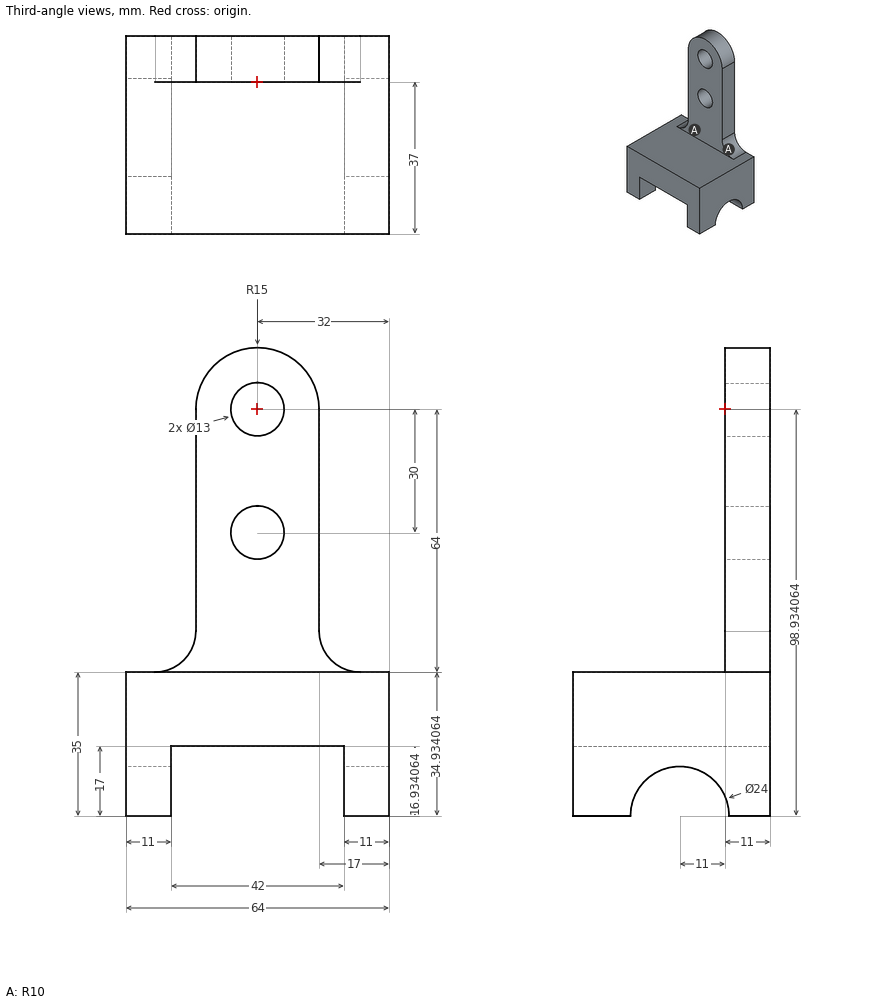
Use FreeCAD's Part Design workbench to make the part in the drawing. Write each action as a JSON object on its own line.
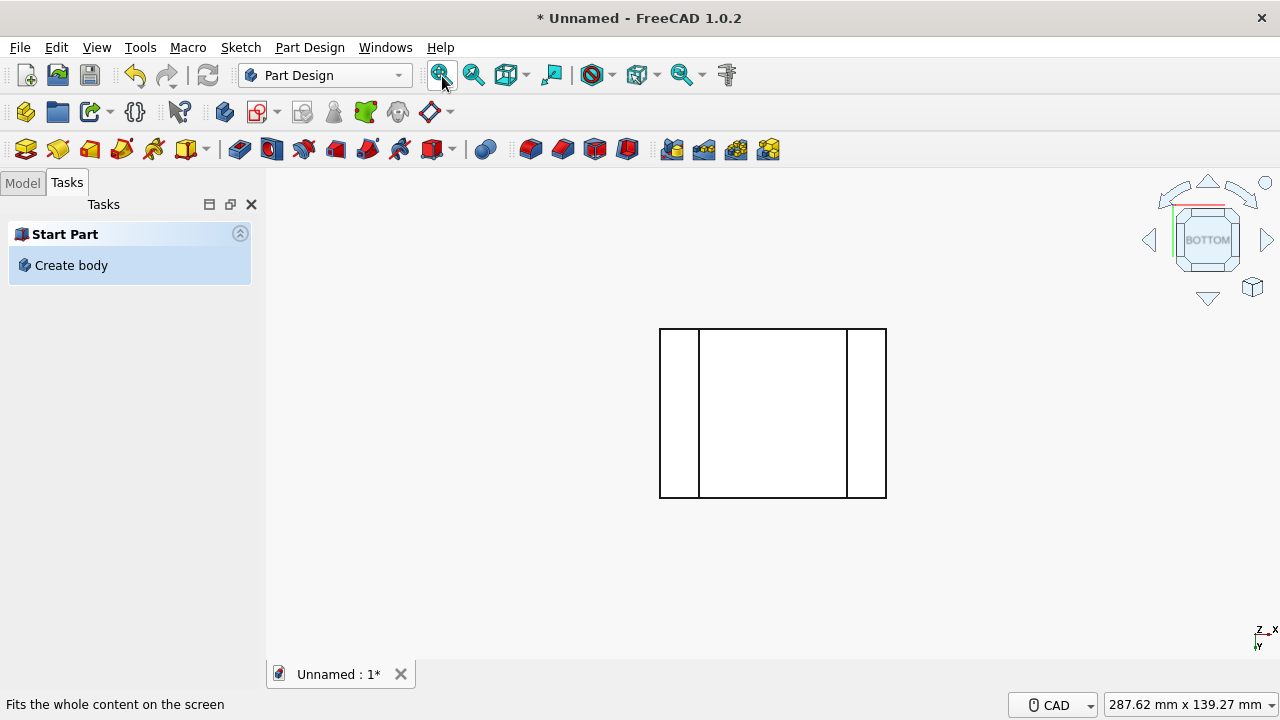
{"action": "key", "text": "4"}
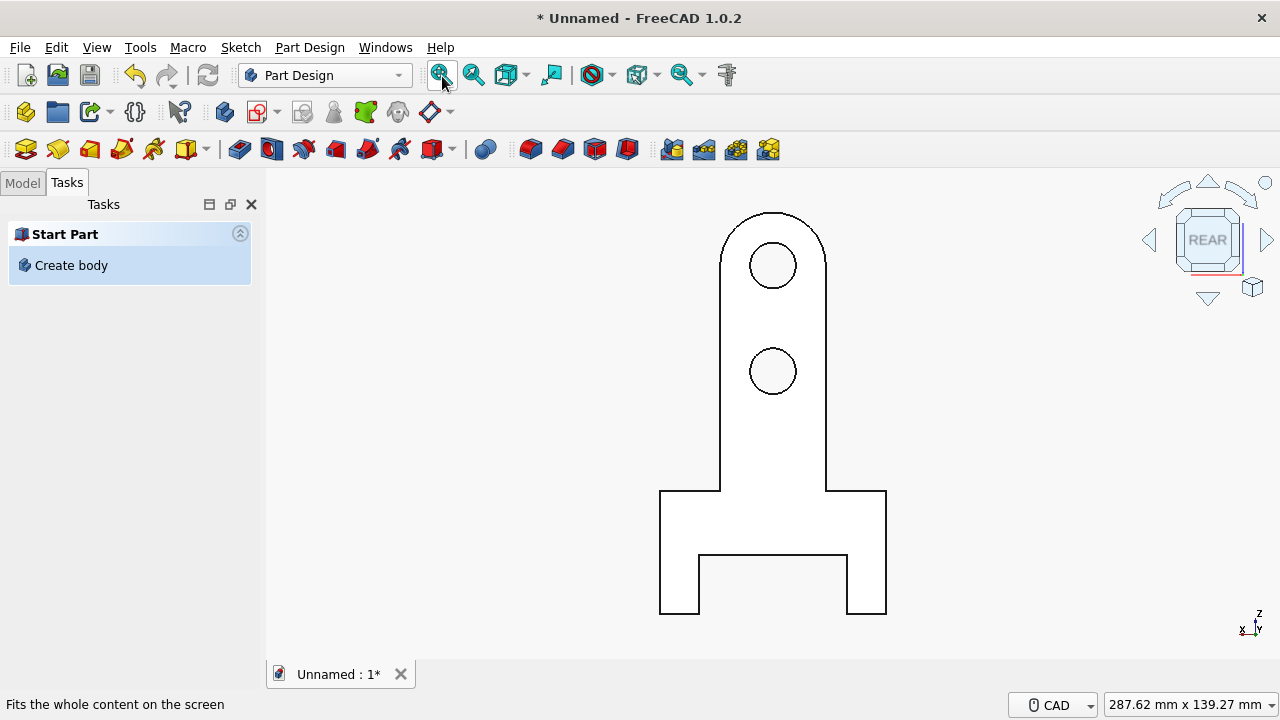
{"action": "key", "text": "6"}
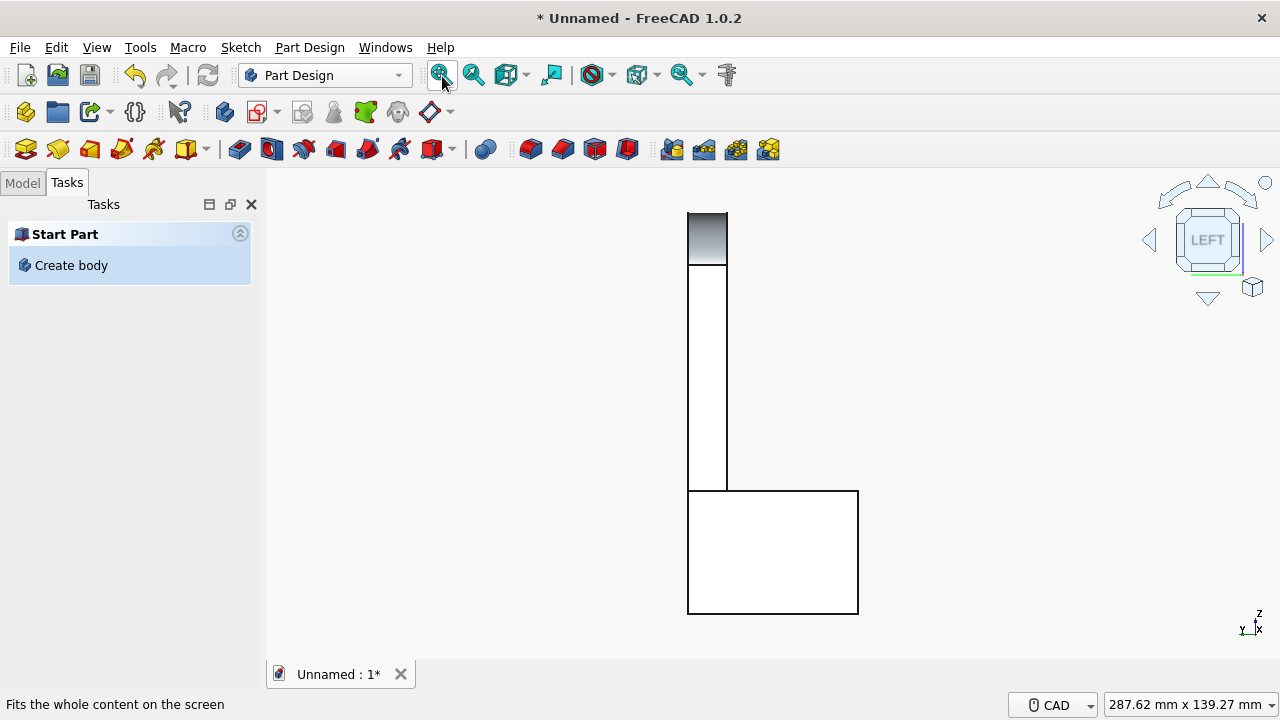
{"action": "key", "text": "v 3"}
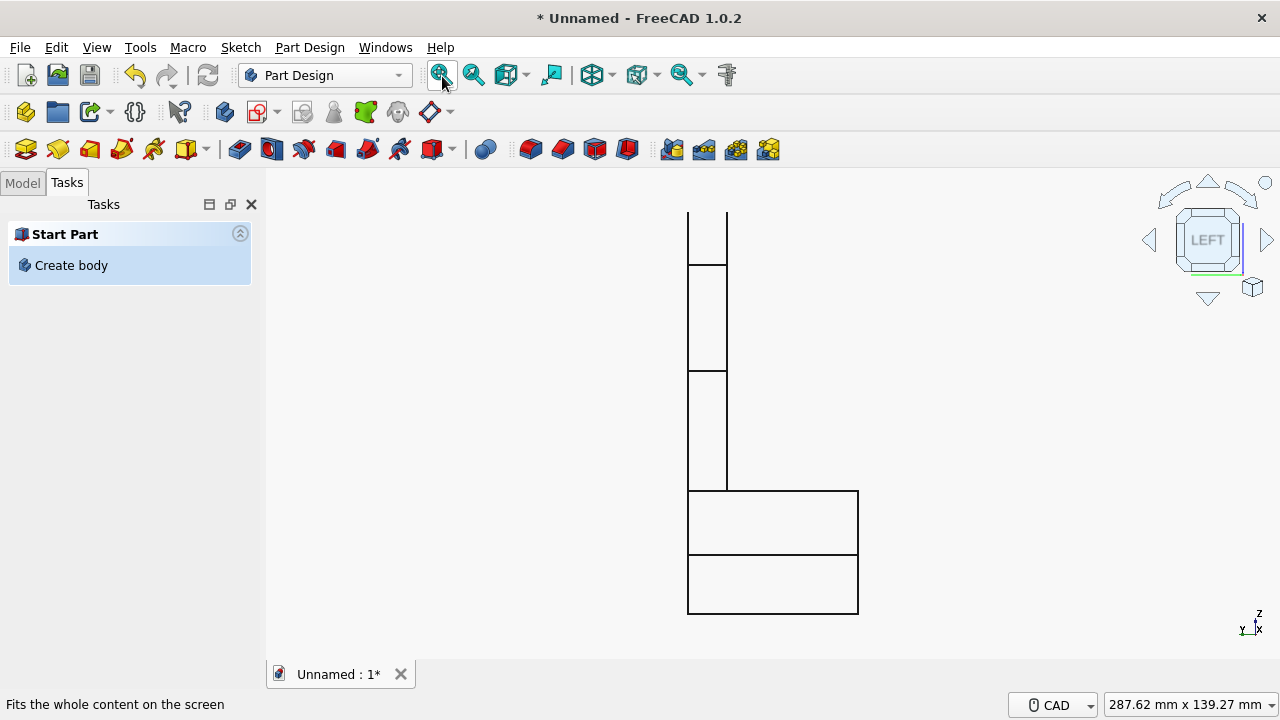
{"action": "key", "text": "0"}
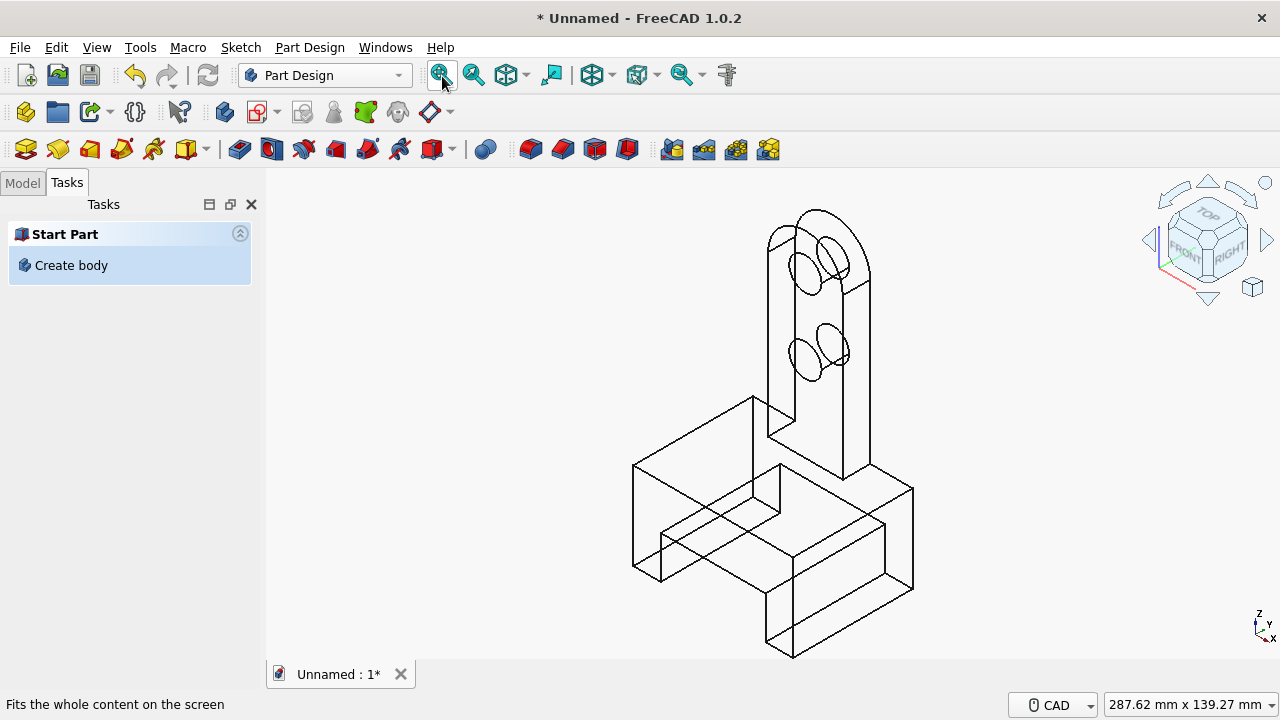
{"action": "left_click", "coordinate": [782, 428]}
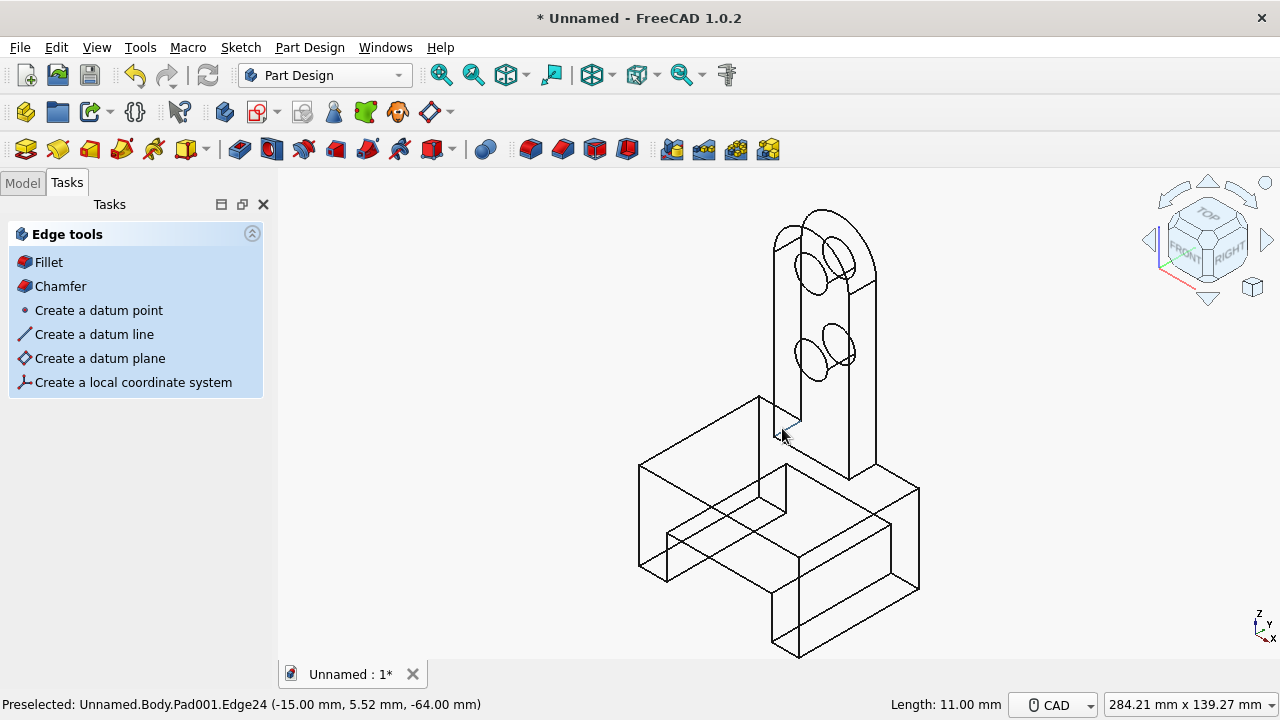
{"action": "left_click", "coordinate": [863, 471], "text": "ctrl"}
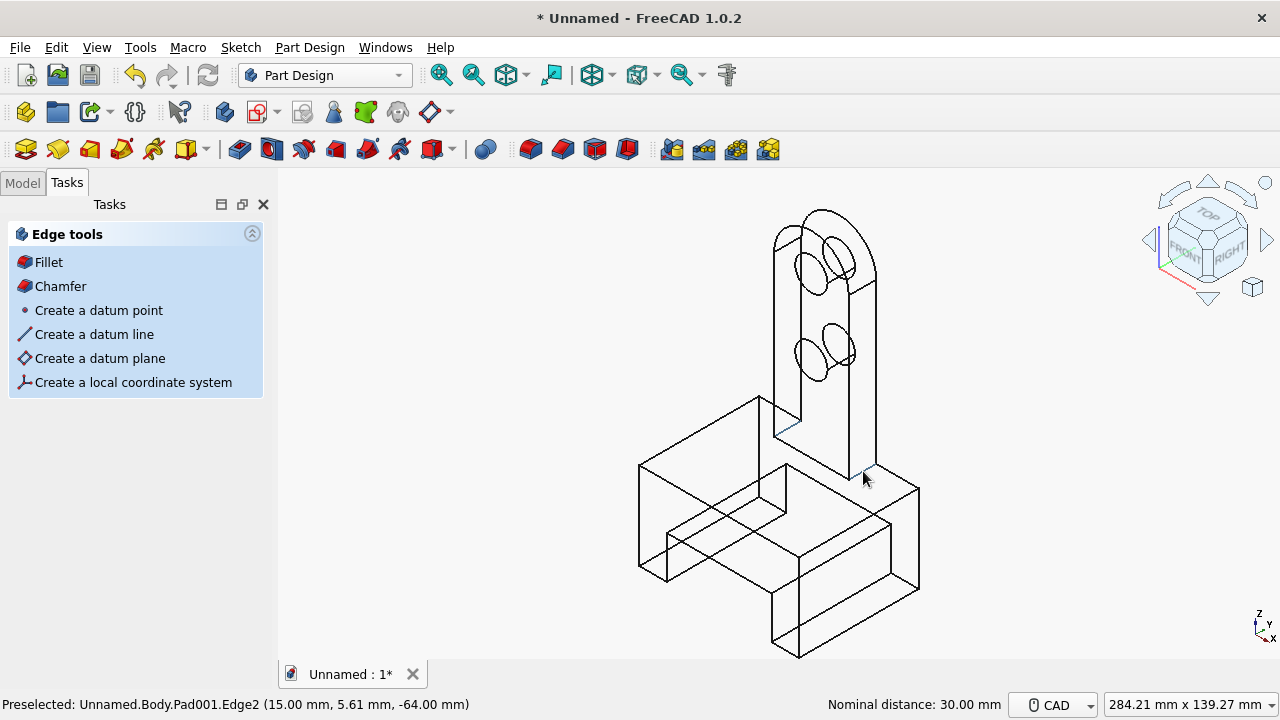
{"action": "key", "text": "v 1"}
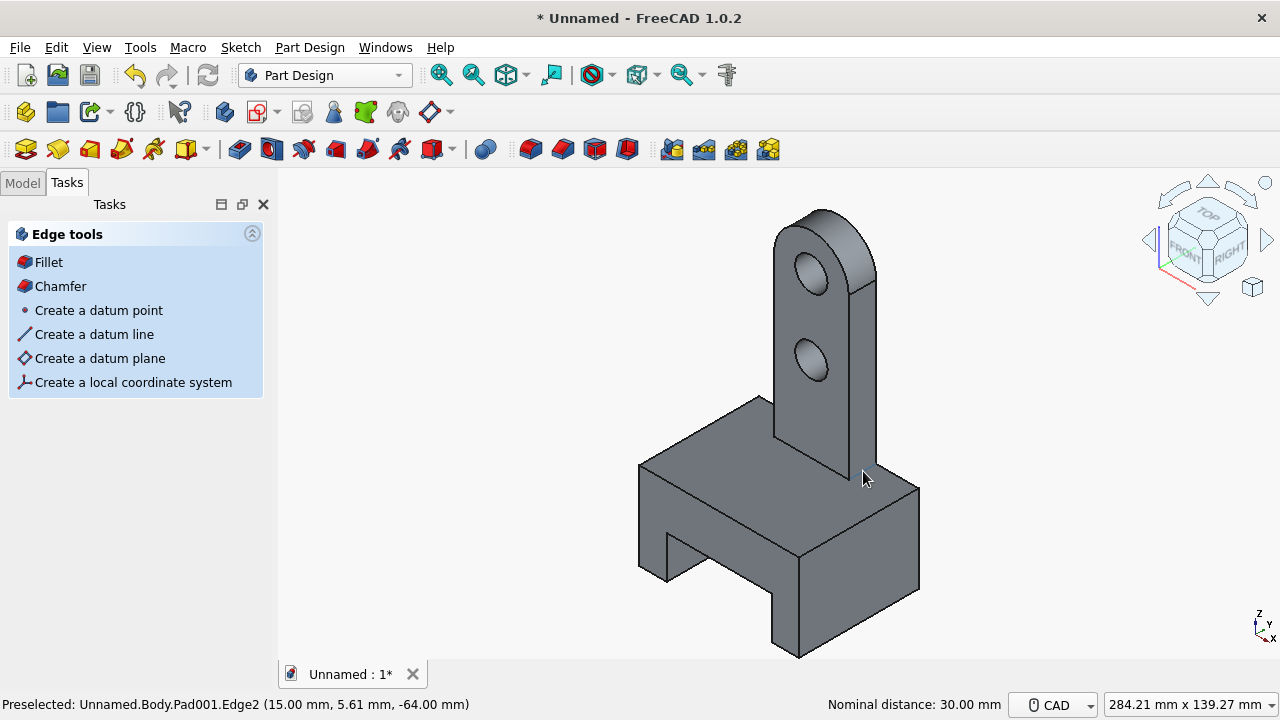
{"action": "left_click", "coordinate": [532, 150]}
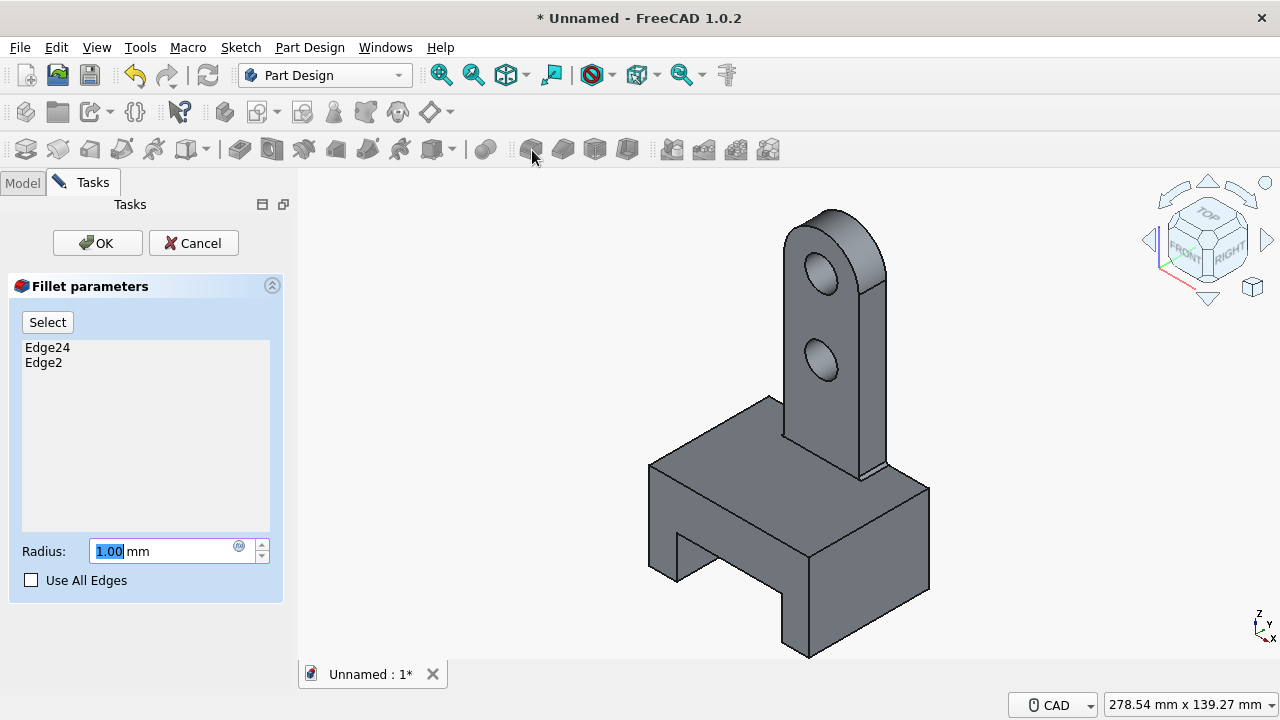
{"action": "type", "text": "10"}
{"action": "key", "text": "Tab"}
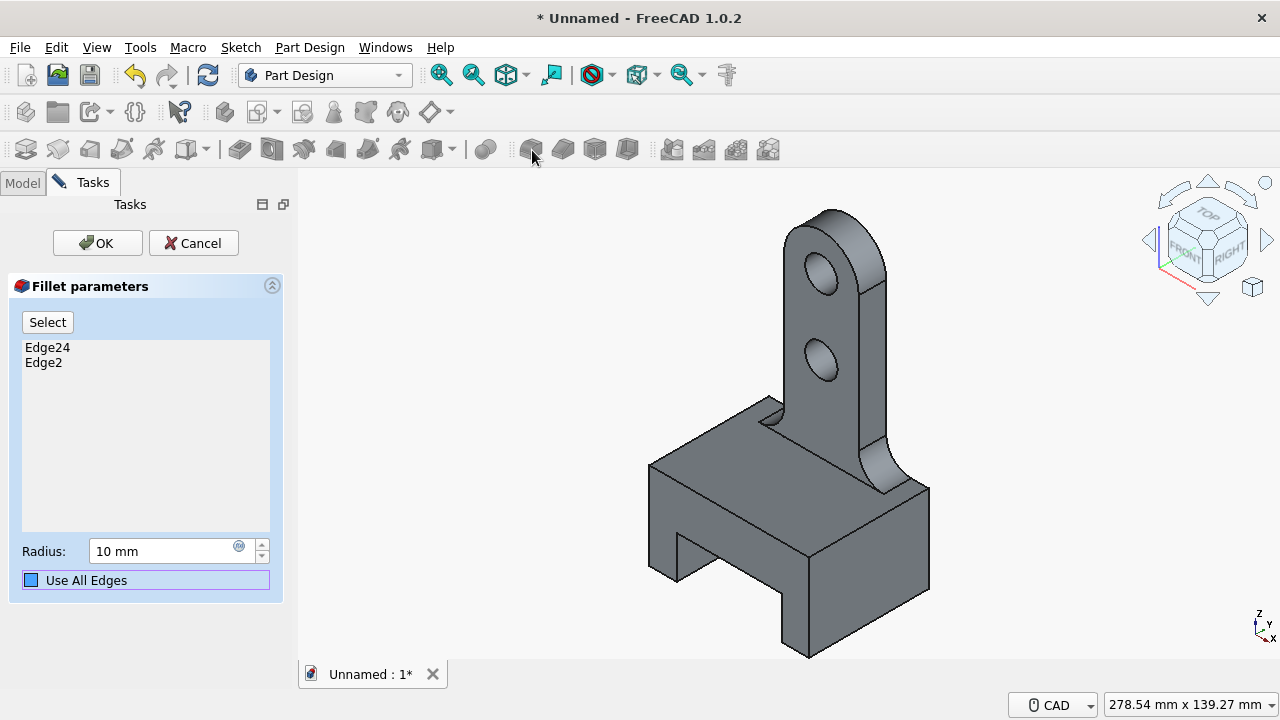
{"action": "left_click", "coordinate": [98, 243]}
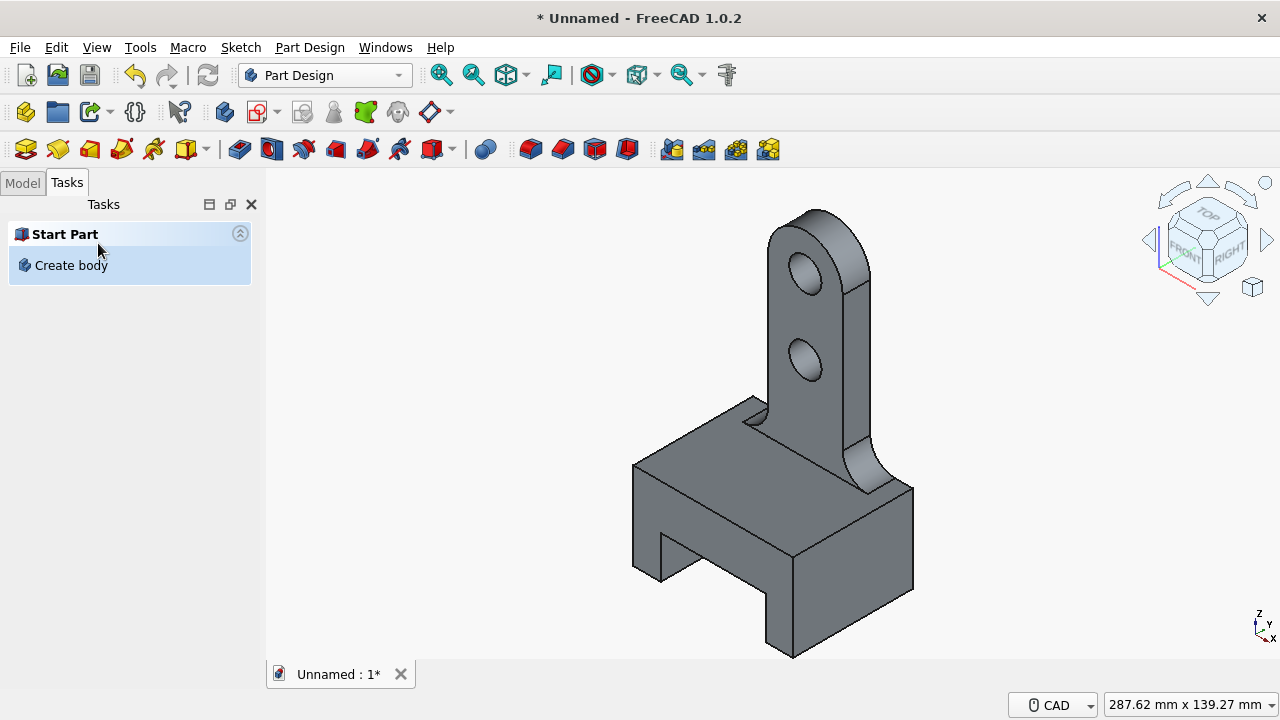
{"action": "left_click", "coordinate": [853, 572]}